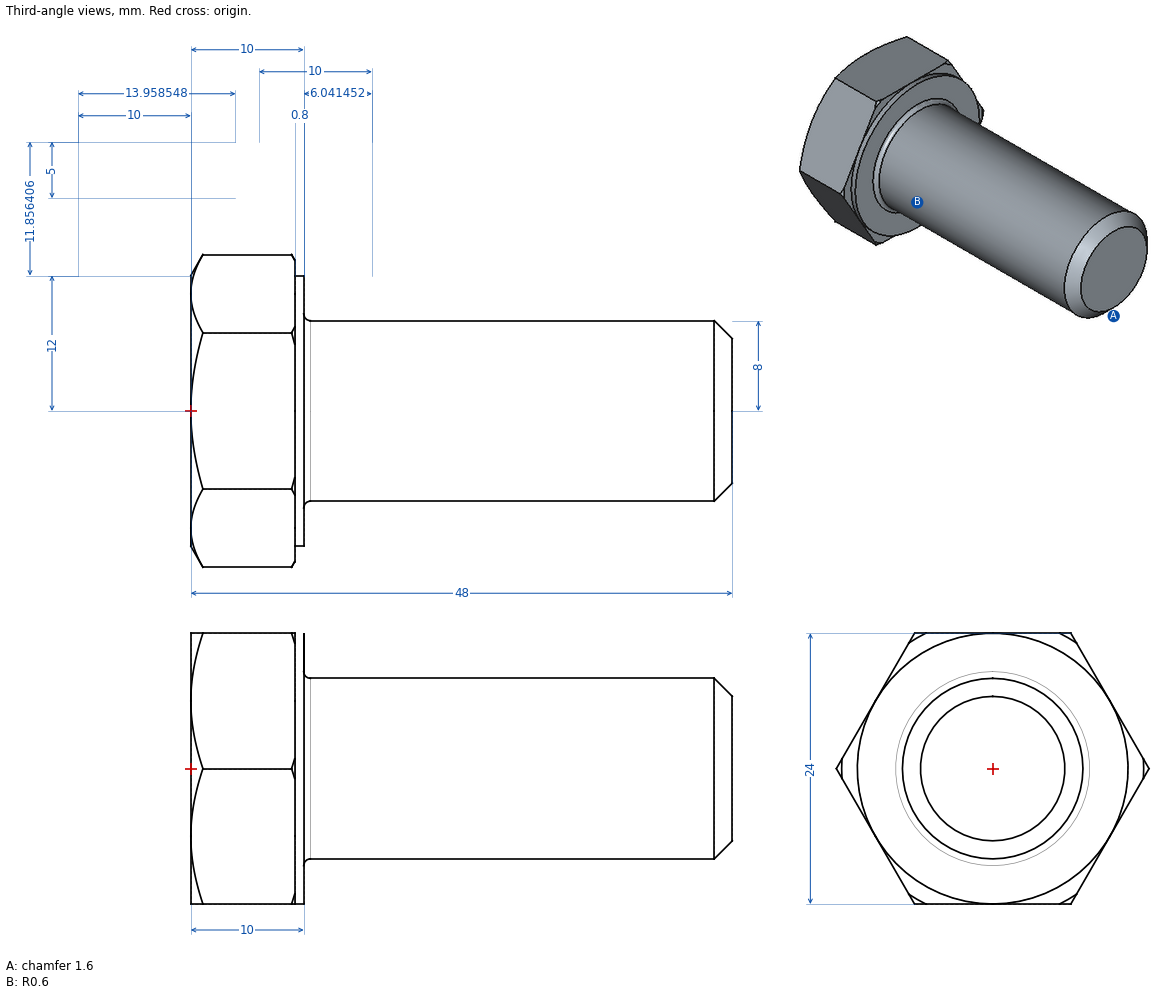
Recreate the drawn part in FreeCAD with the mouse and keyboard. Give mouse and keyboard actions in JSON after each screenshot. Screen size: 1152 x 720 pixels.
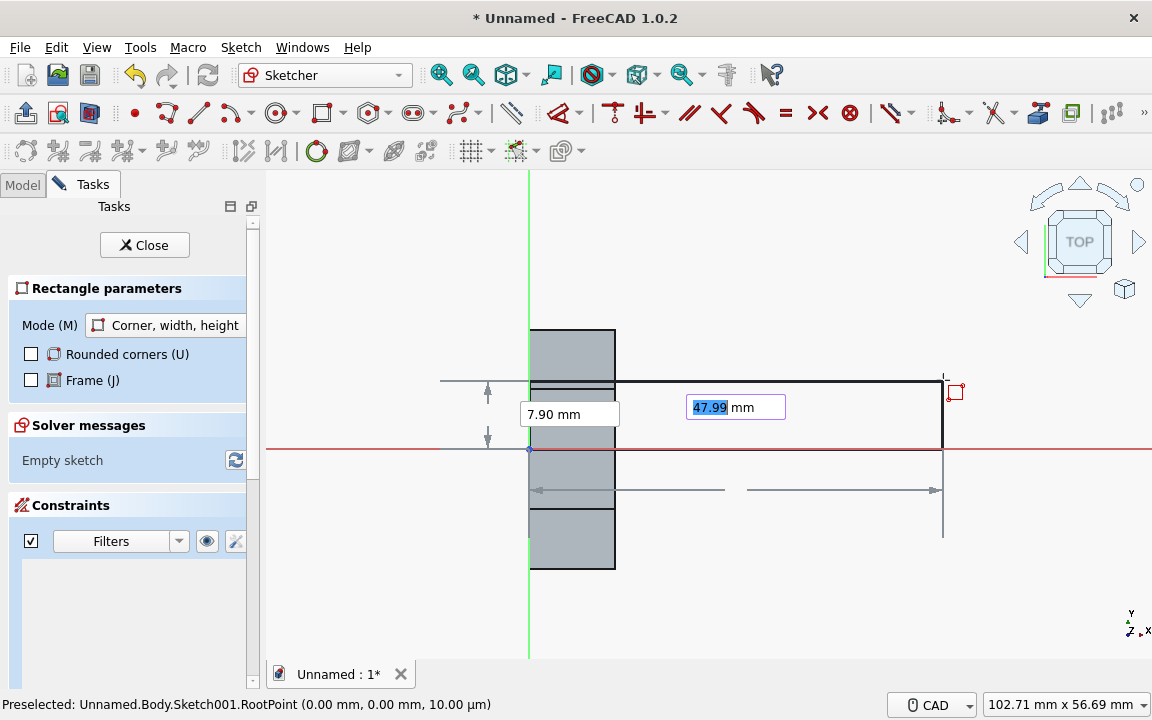
{"action": "type", "text": "48"}
{"action": "key", "text": "Tab"}
{"action": "type", "text": "8"}
{"action": "key", "text": "Return"}
{"action": "key", "text": "Escape"}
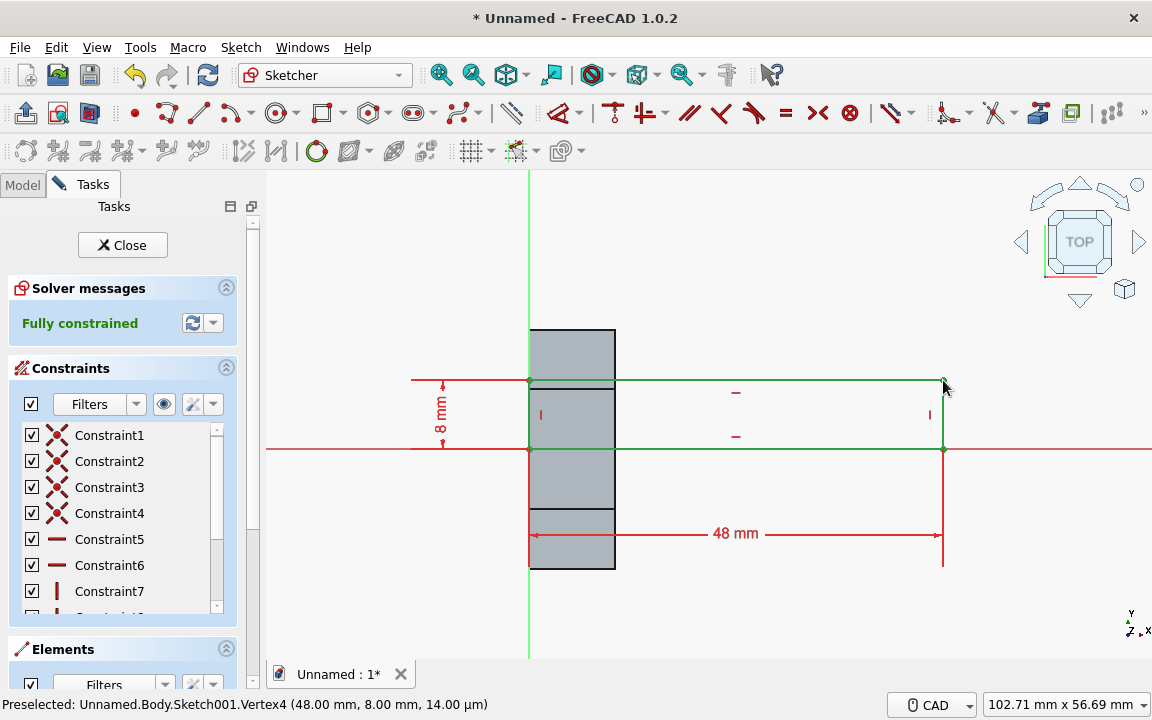
{"action": "left_click", "coordinate": [123, 245]}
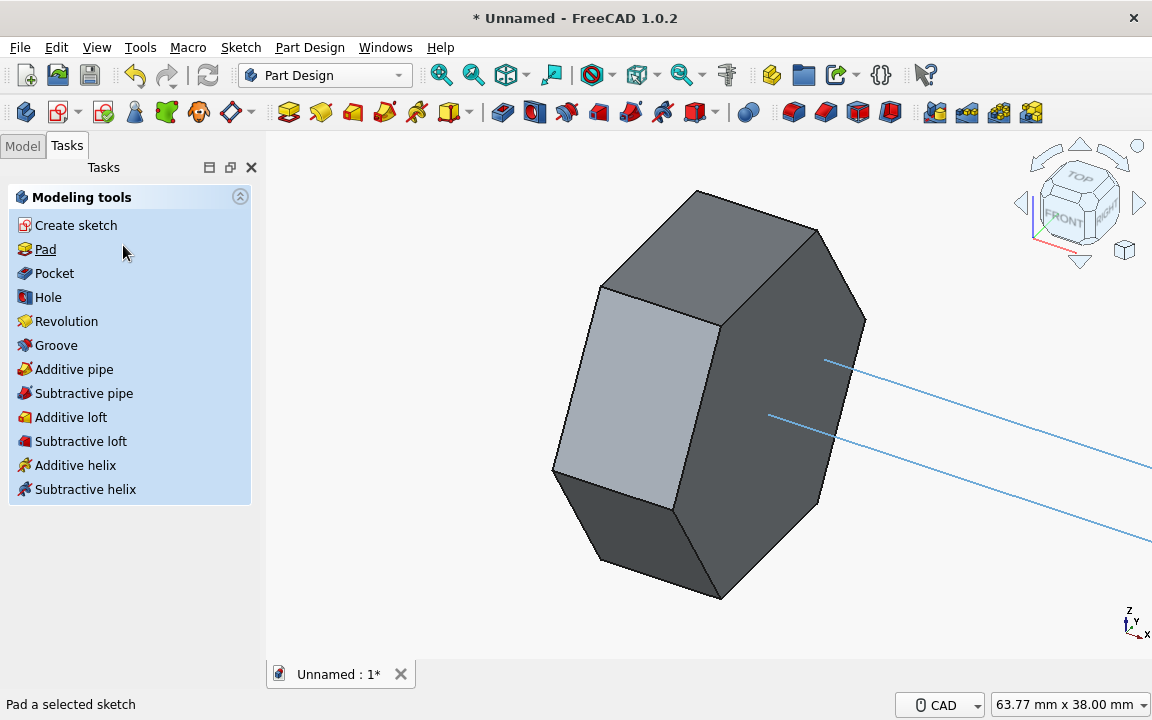
{"action": "left_click", "coordinate": [322, 112]}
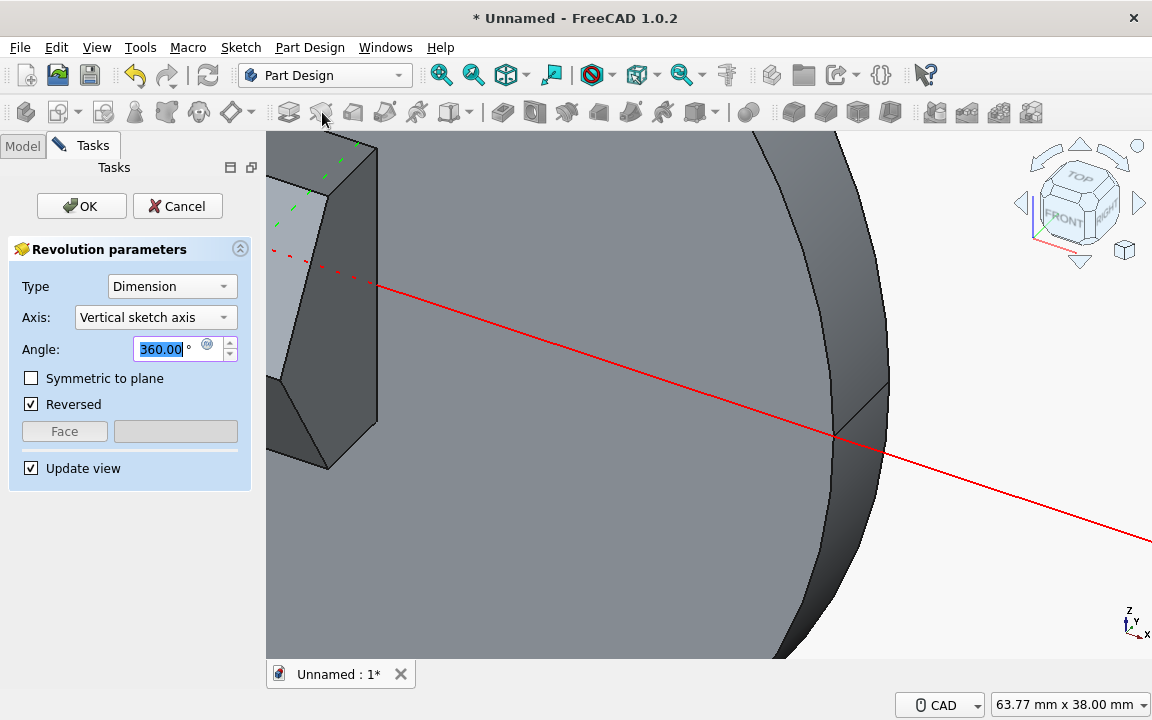
{"action": "left_click", "coordinate": [156, 318]}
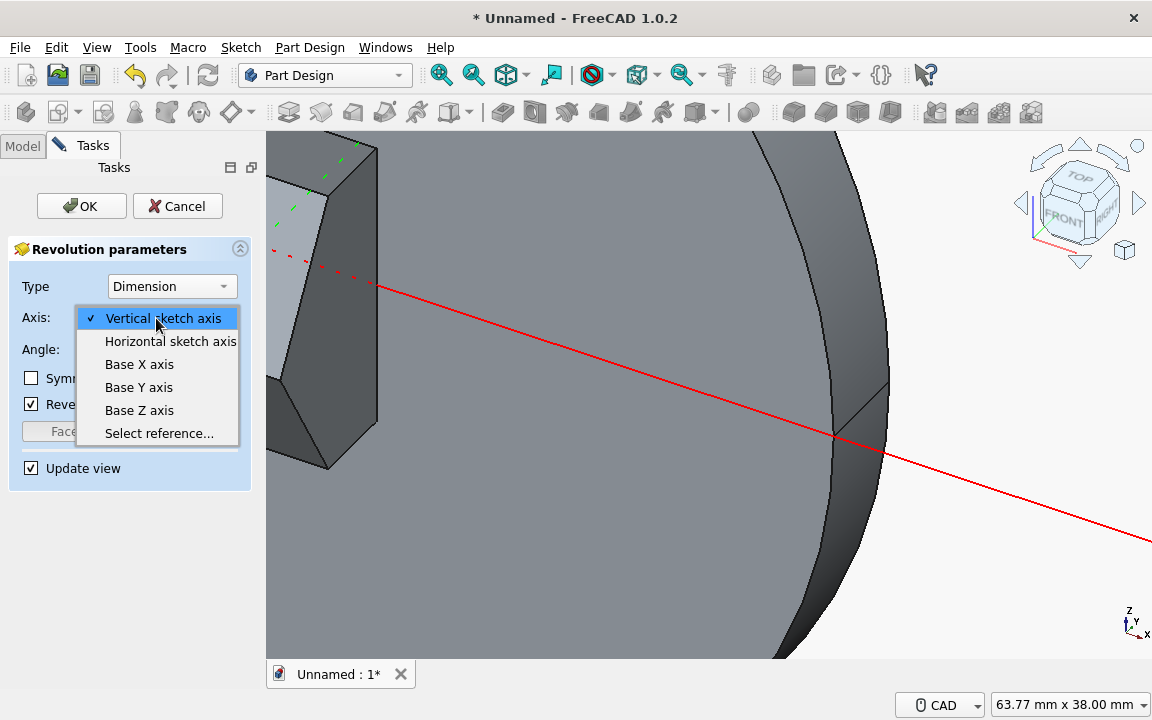
{"action": "left_click", "coordinate": [156, 342]}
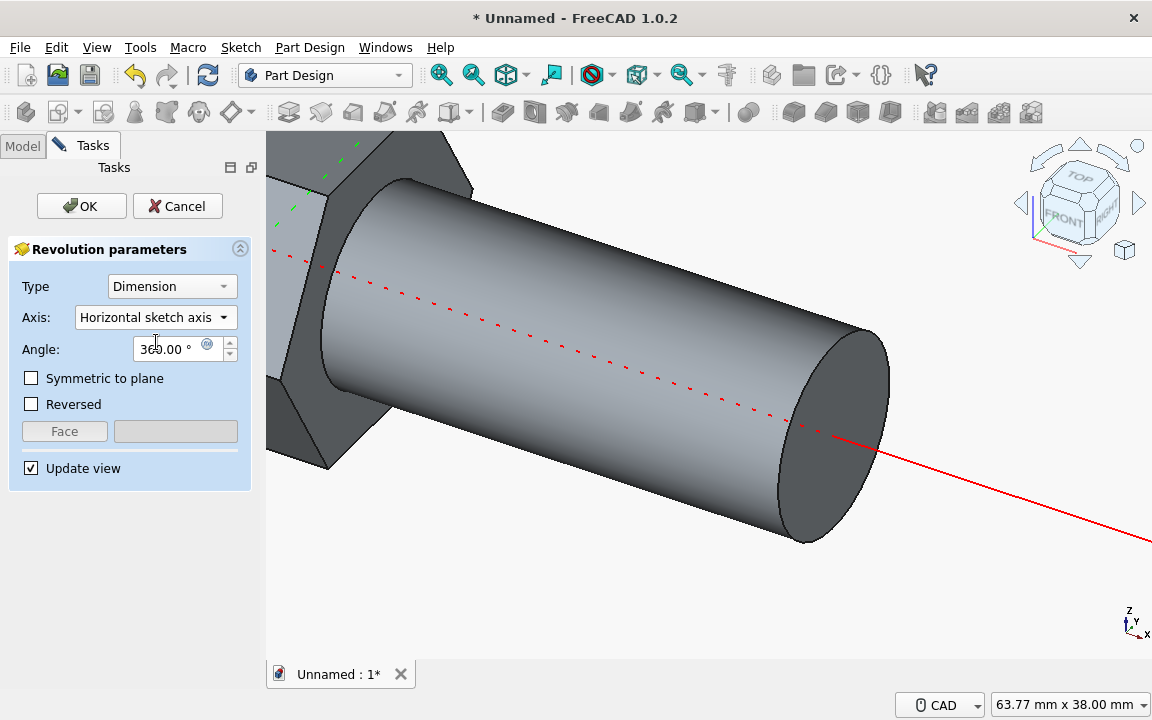
{"action": "left_click", "coordinate": [82, 206]}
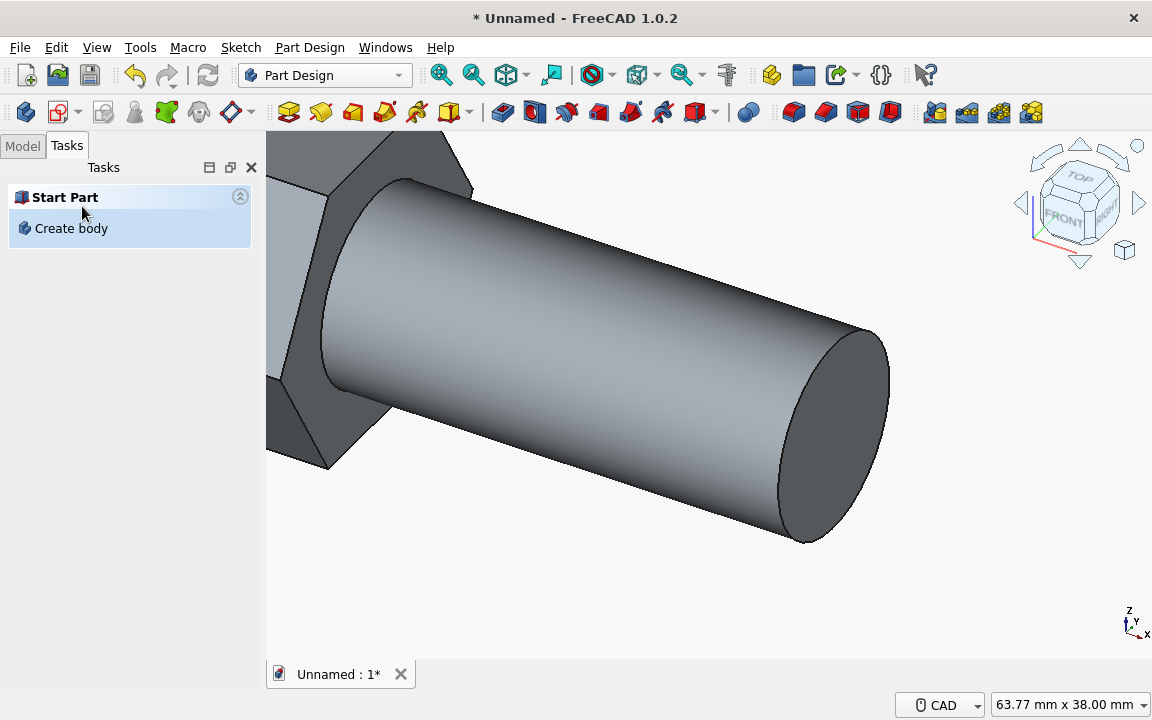
{"action": "left_click", "coordinate": [442, 76]}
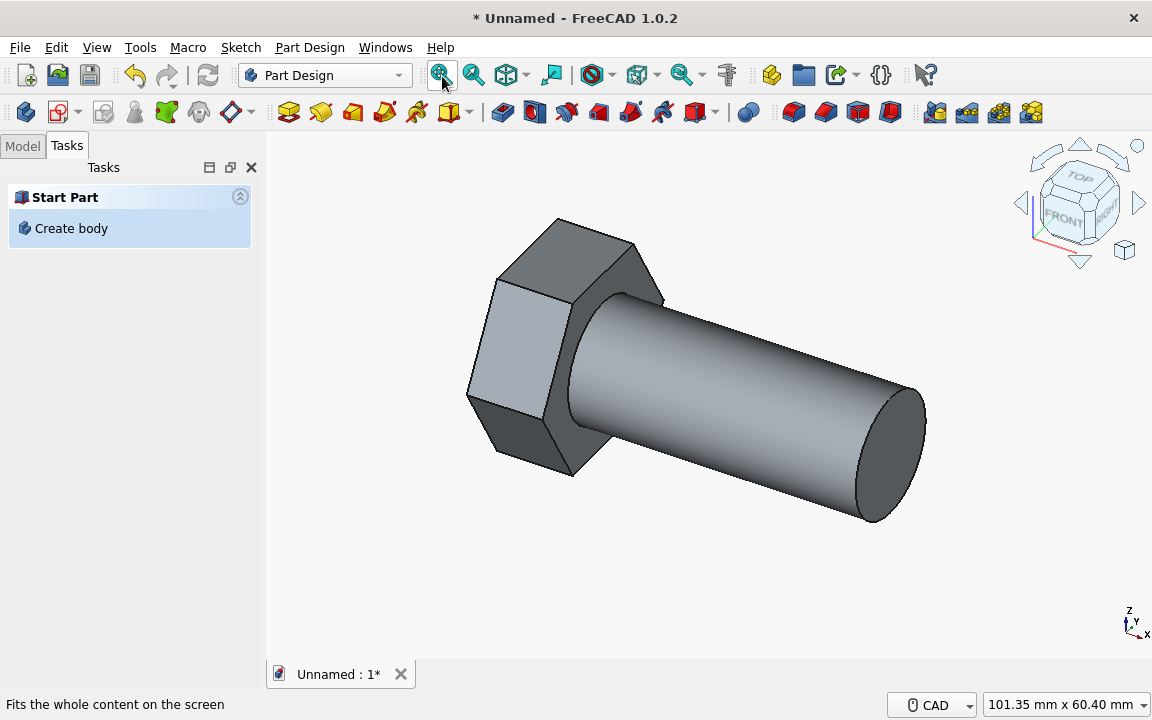
{"action": "left_click", "coordinate": [58, 112]}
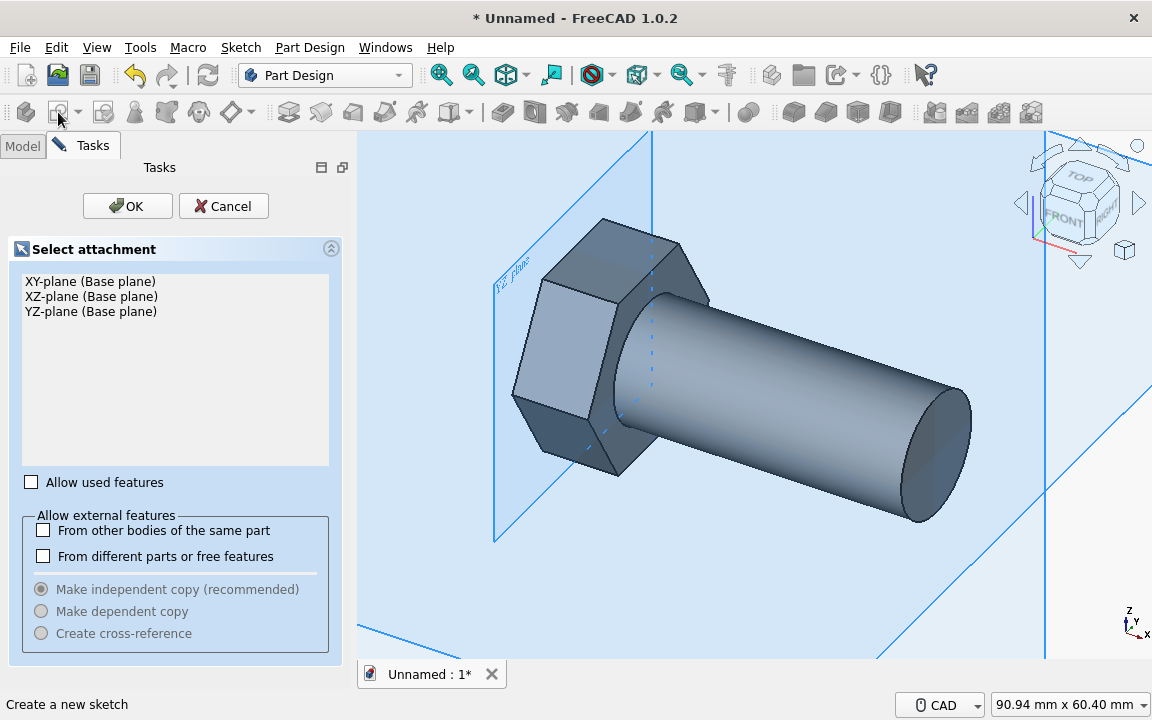
{"action": "left_click", "coordinate": [82, 282]}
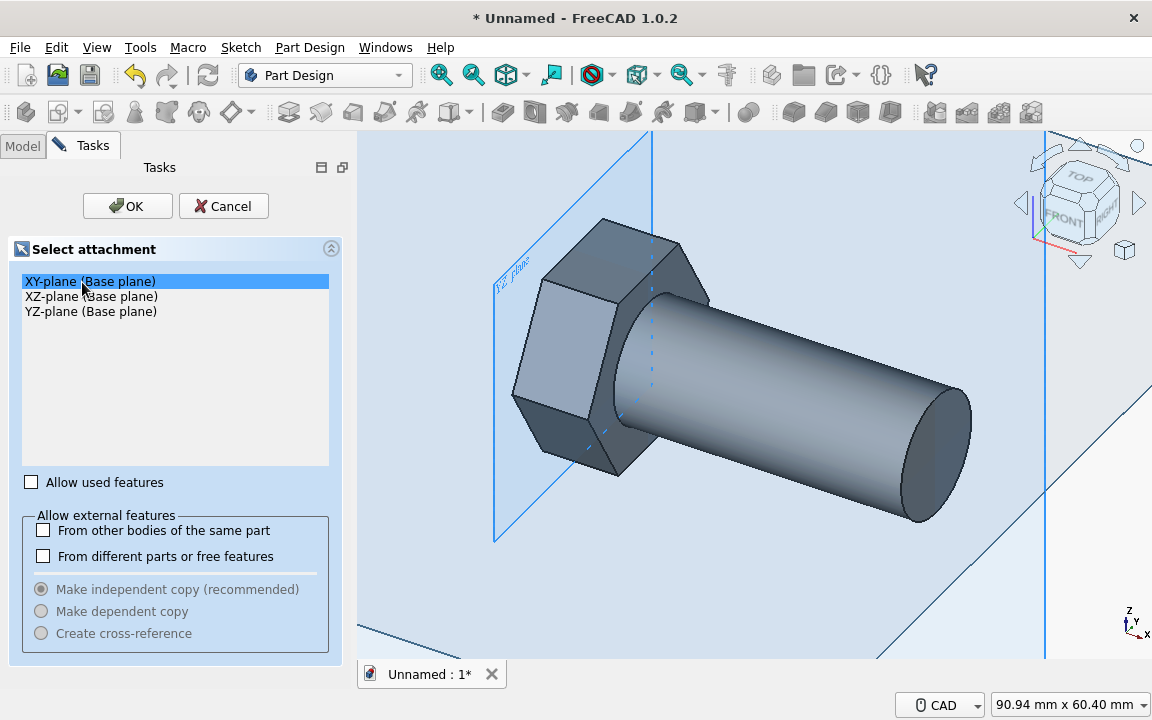
{"action": "left_click", "coordinate": [128, 206]}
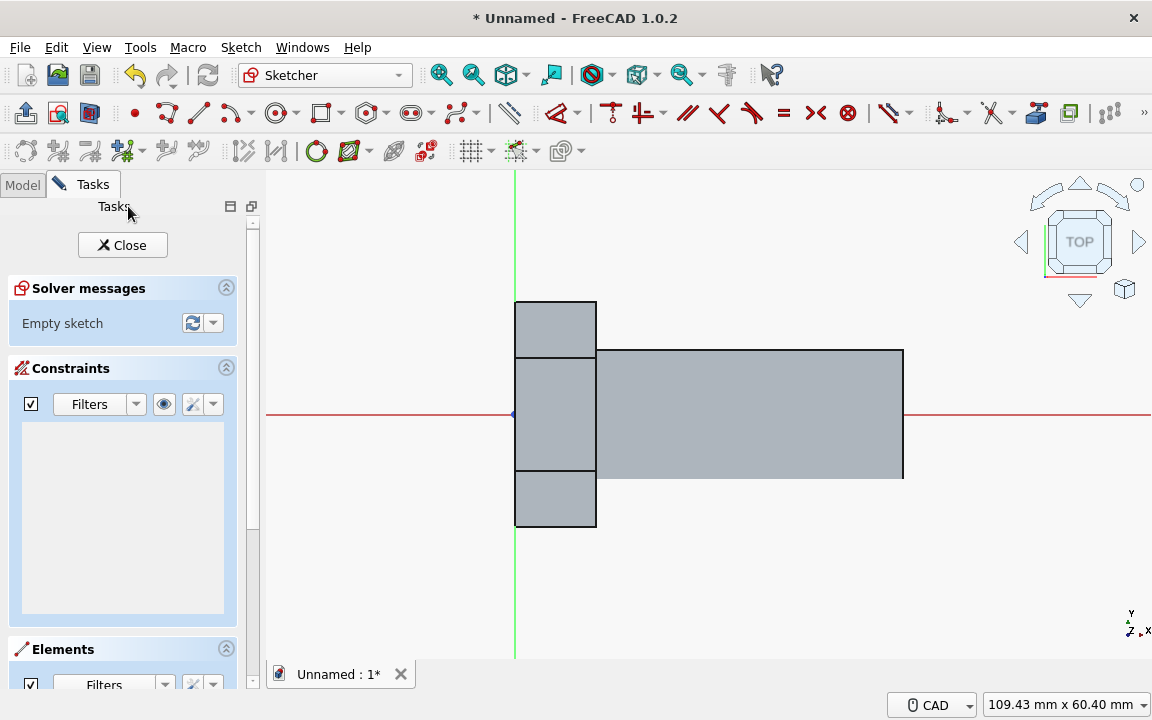
{"action": "left_click", "coordinate": [90, 114]}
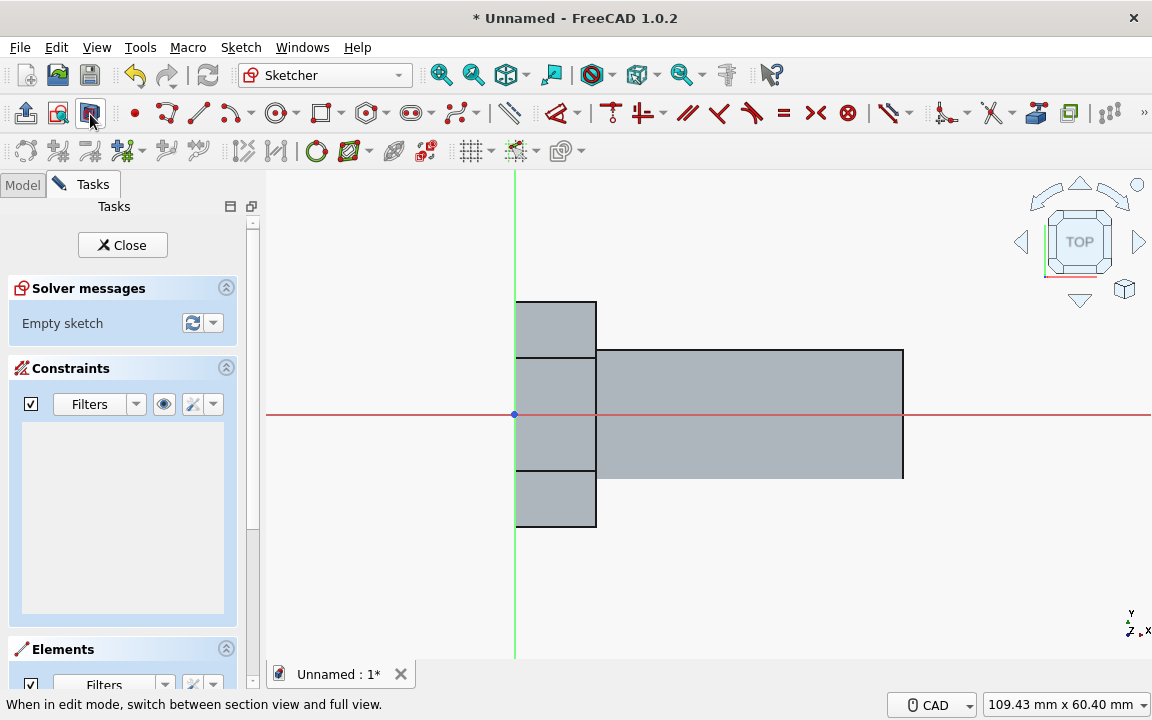
{"action": "scroll", "coordinate": [294, 198], "scroll_direction": "up", "scroll_amount": 2}